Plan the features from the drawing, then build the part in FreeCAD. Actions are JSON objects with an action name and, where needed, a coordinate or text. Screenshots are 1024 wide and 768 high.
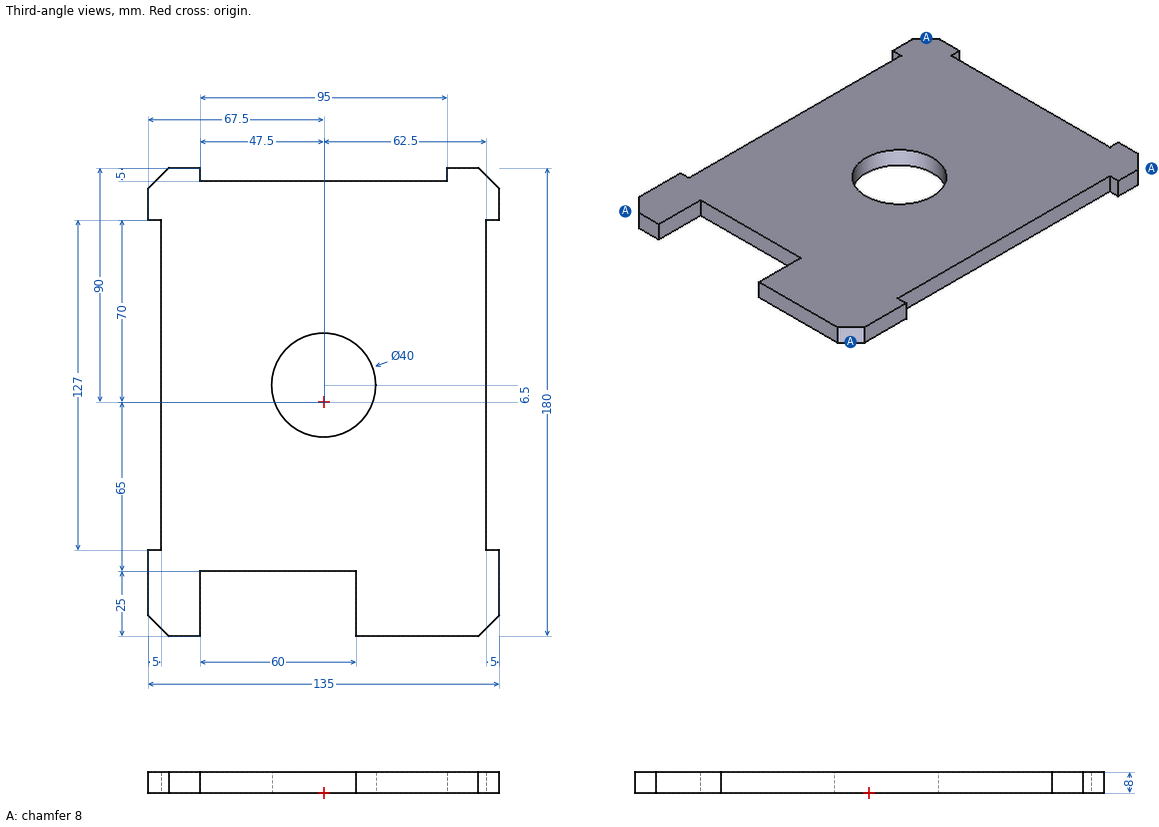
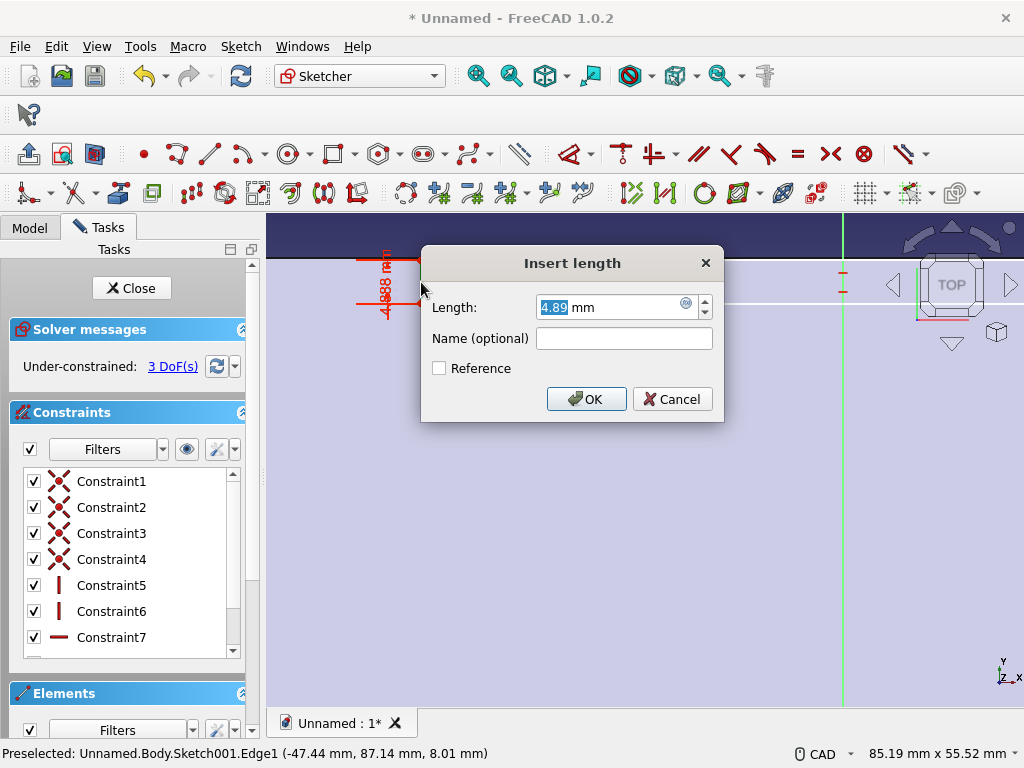
{"action": "type", "text": "5"}
{"action": "key", "text": "Return"}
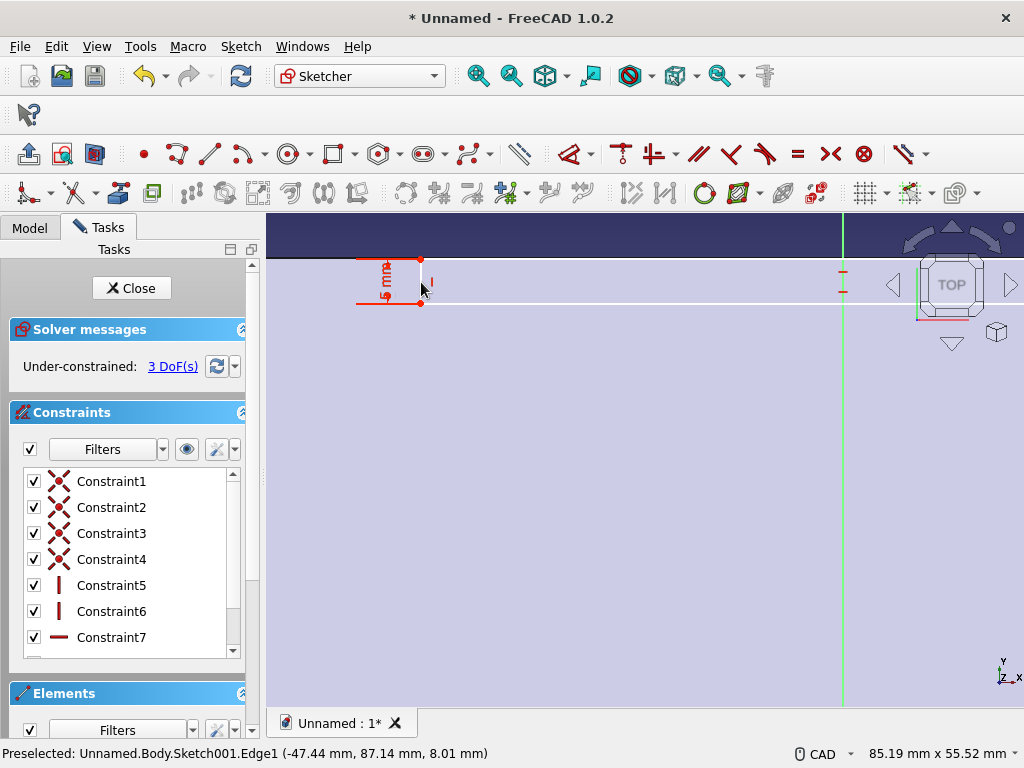
{"action": "left_click", "coordinate": [674, 304]}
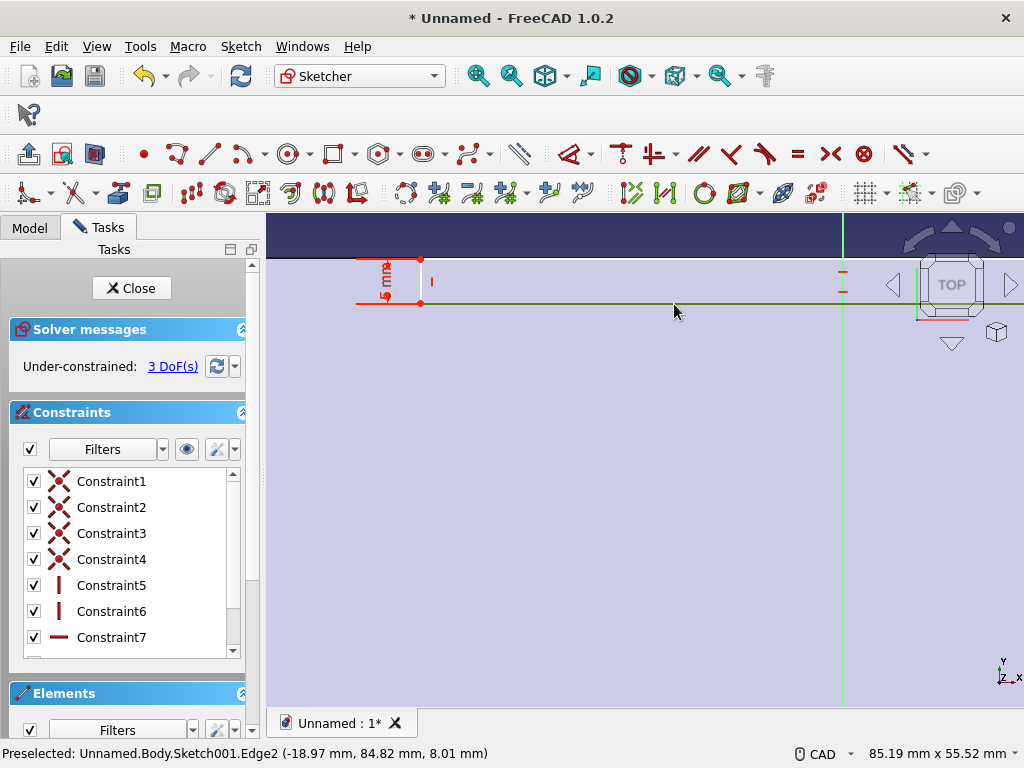
{"action": "key", "text": "l"}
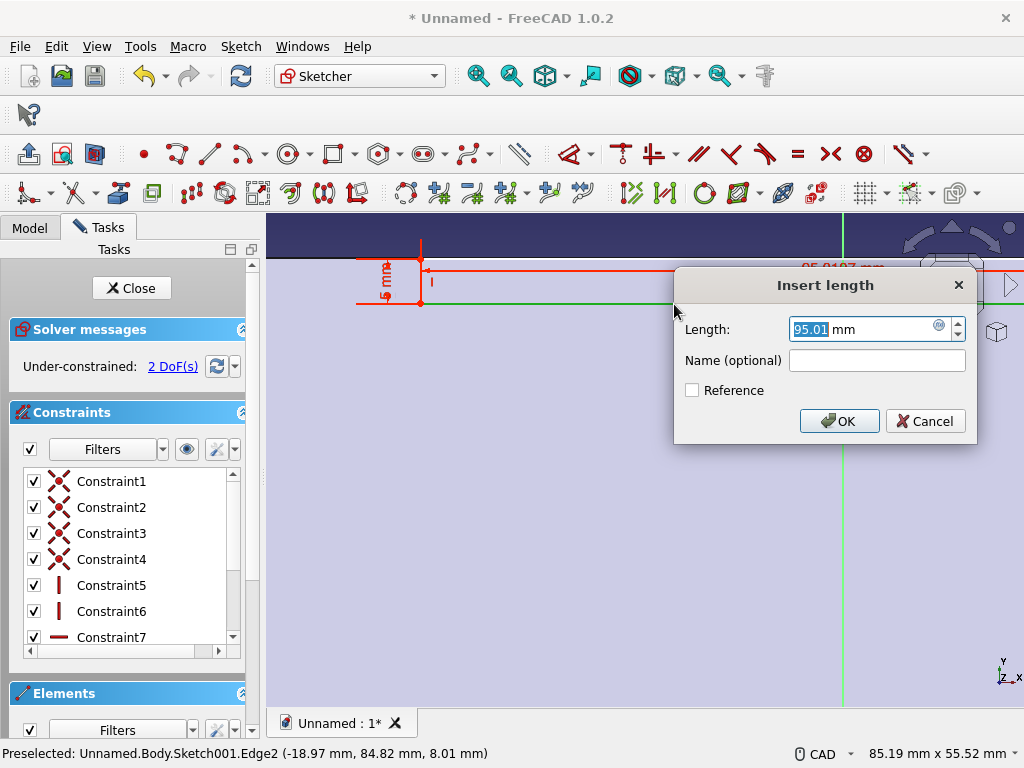
{"action": "type", "text": "95"}
{"action": "key", "text": "Return"}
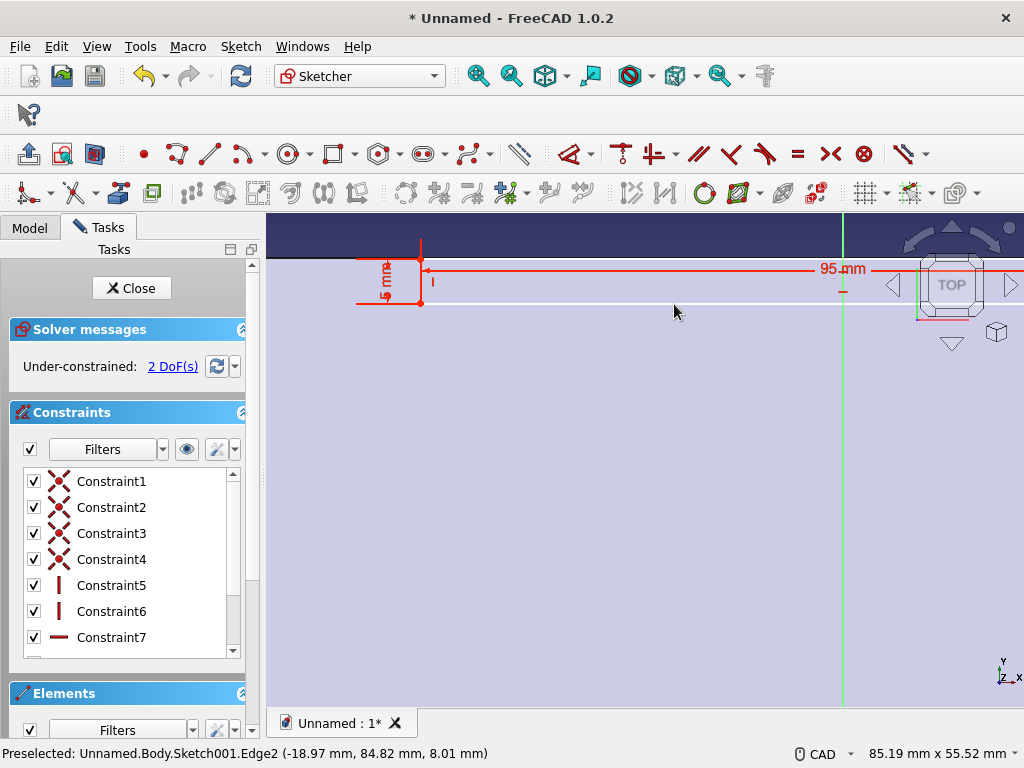
{"action": "left_click", "coordinate": [421, 259]}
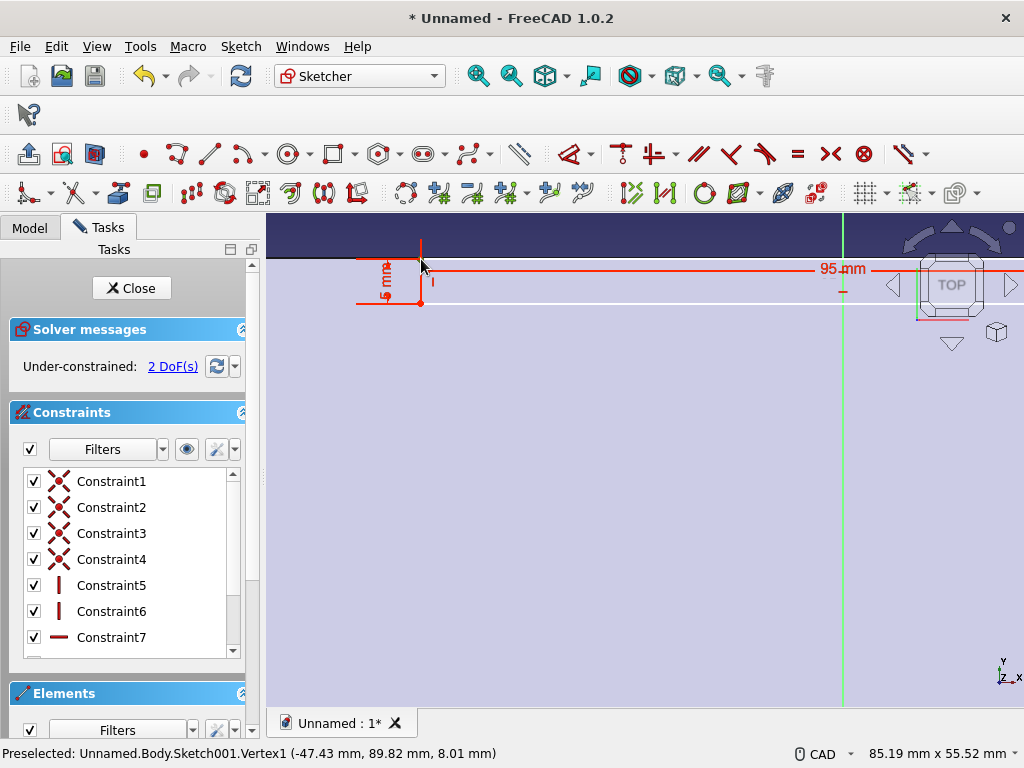
{"action": "left_click", "coordinate": [590, 154]}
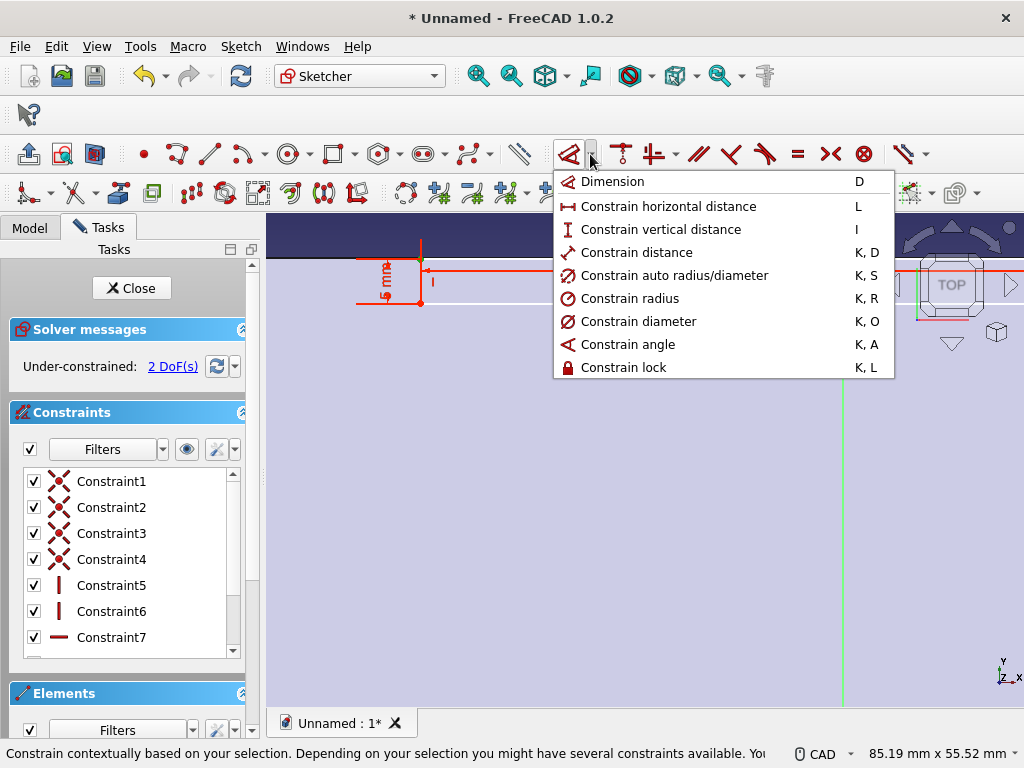
{"action": "left_click", "coordinate": [724, 230]}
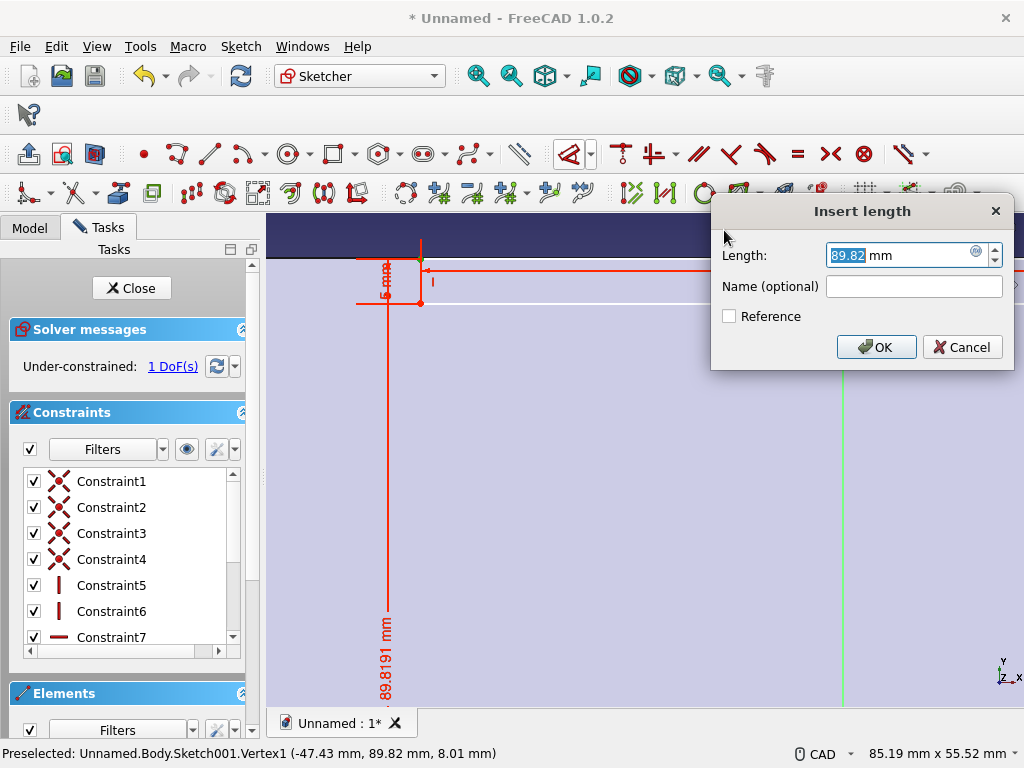
{"action": "type", "text": "90"}
{"action": "key", "text": "Return"}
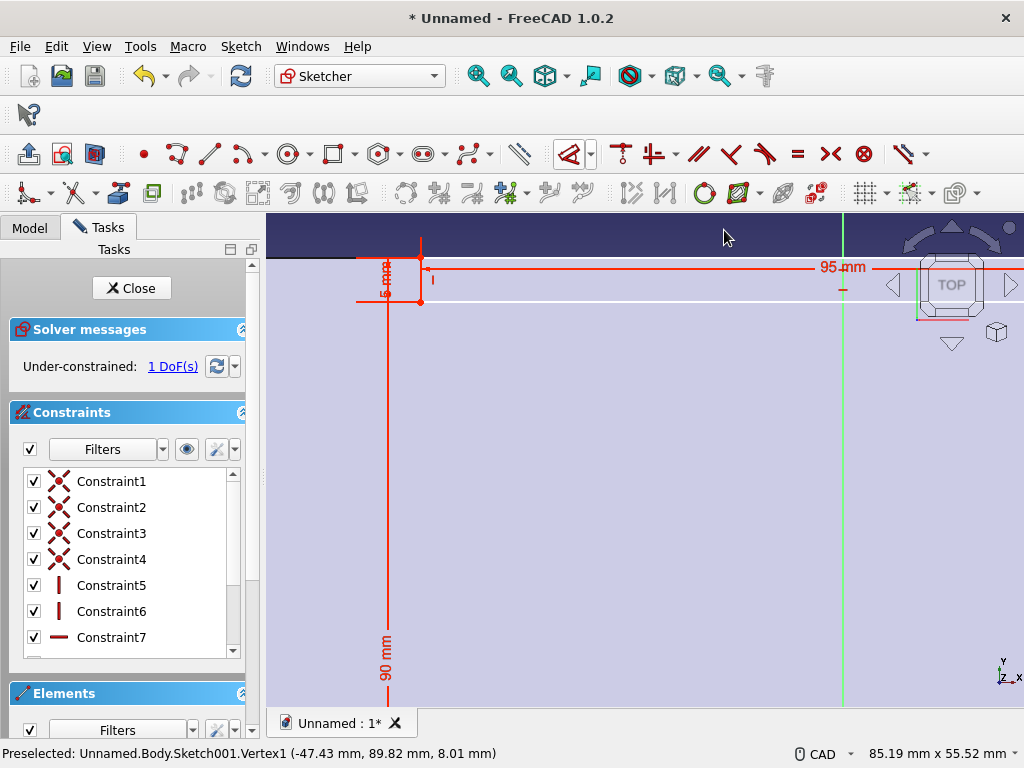
{"action": "left_click", "coordinate": [421, 258]}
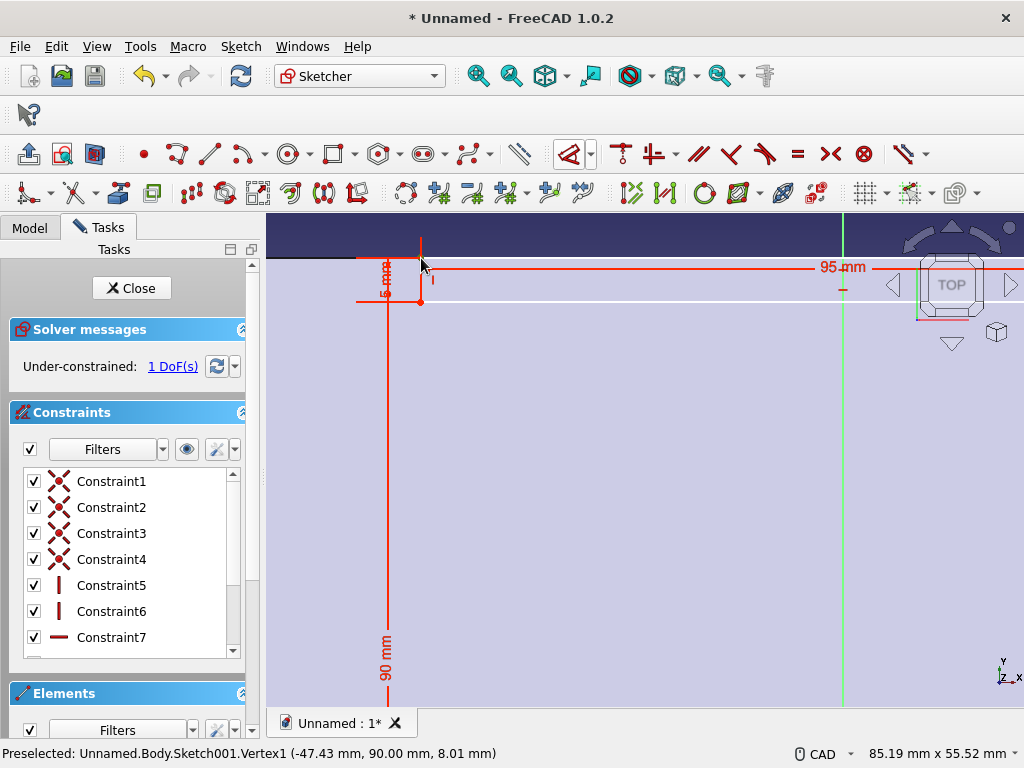
{"action": "key", "text": "l"}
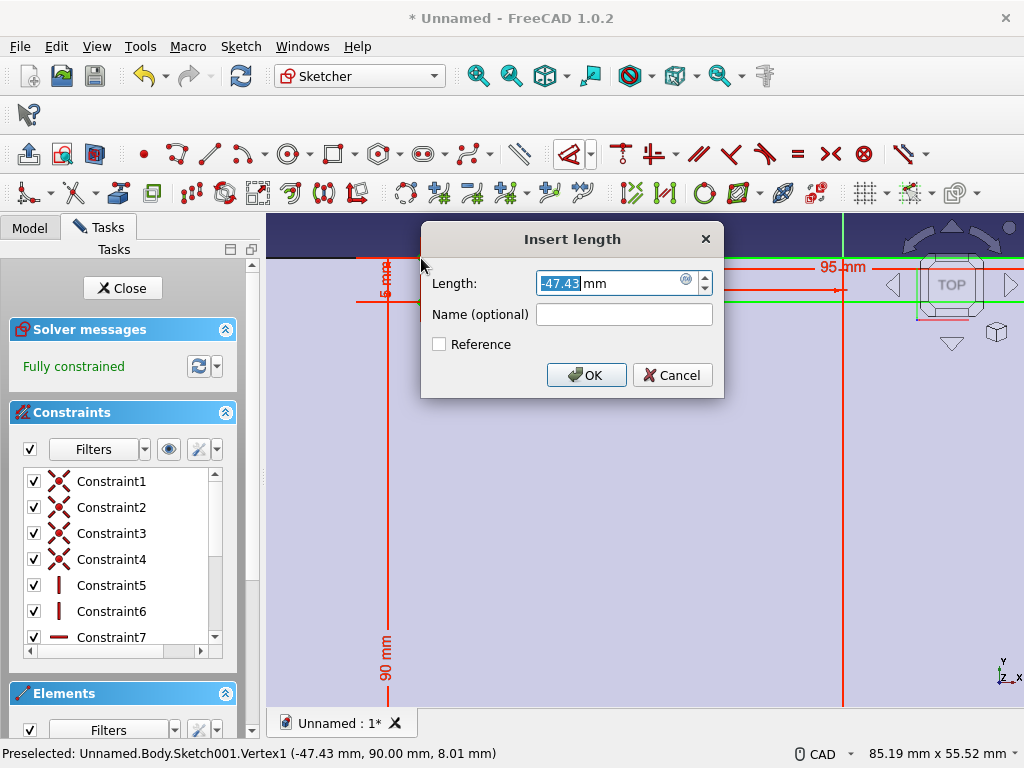
{"action": "type", "text": "-47.5"}
{"action": "key", "text": "Return"}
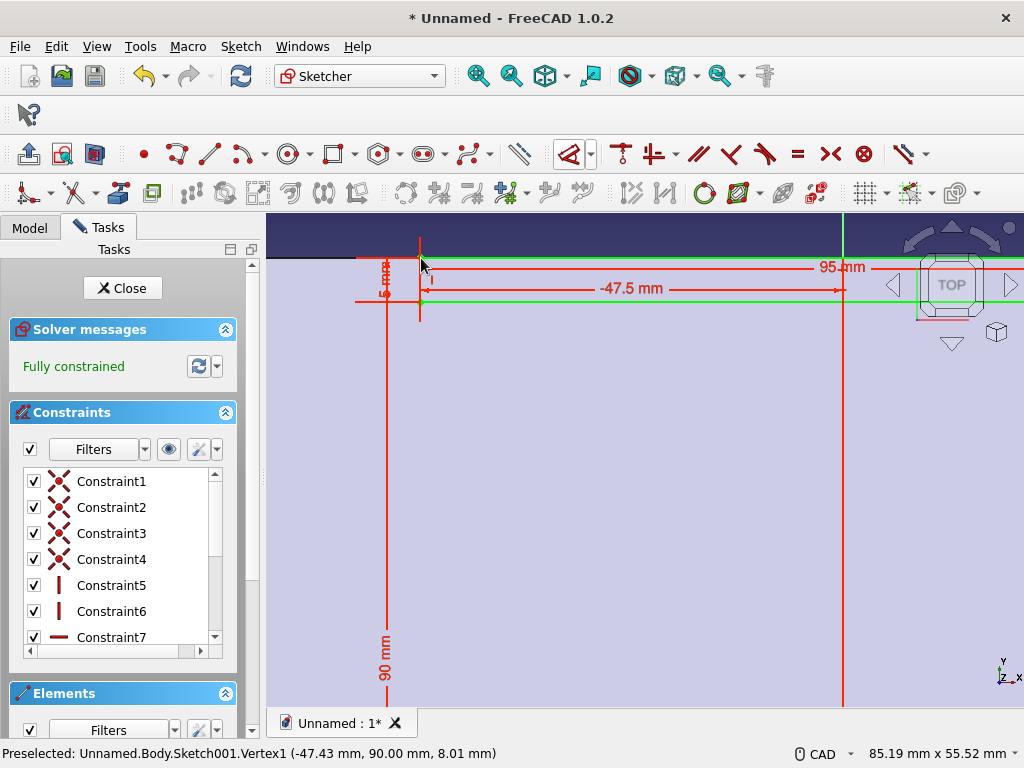
{"action": "left_click", "coordinate": [123, 288]}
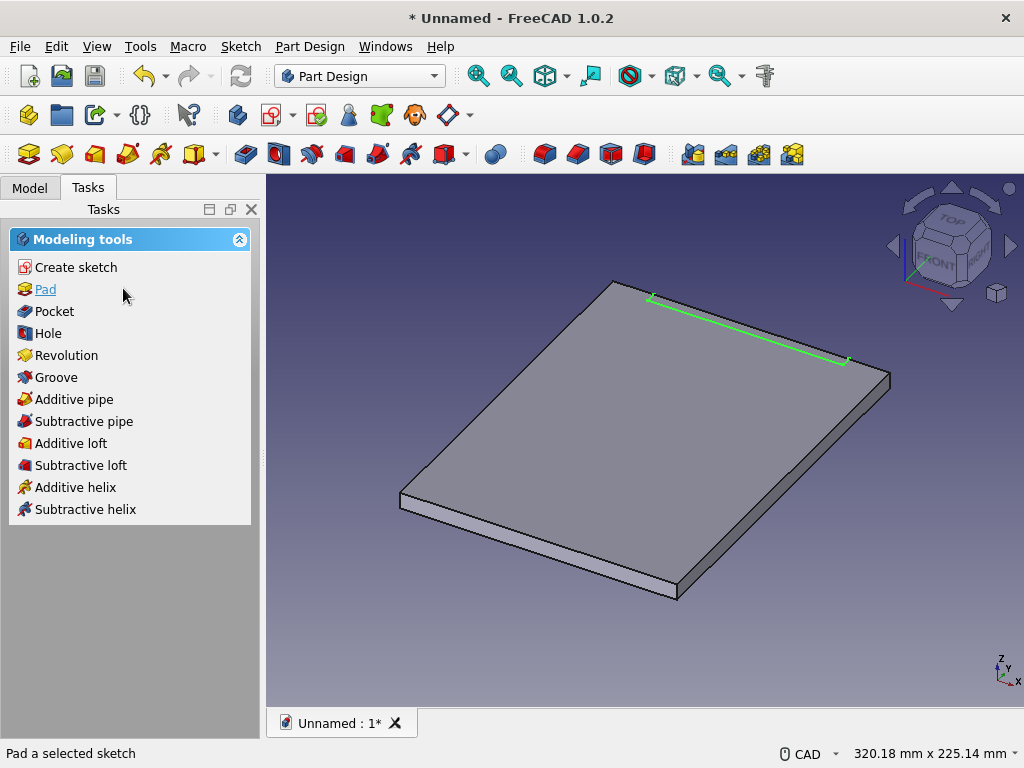
{"action": "left_click", "coordinate": [246, 154]}